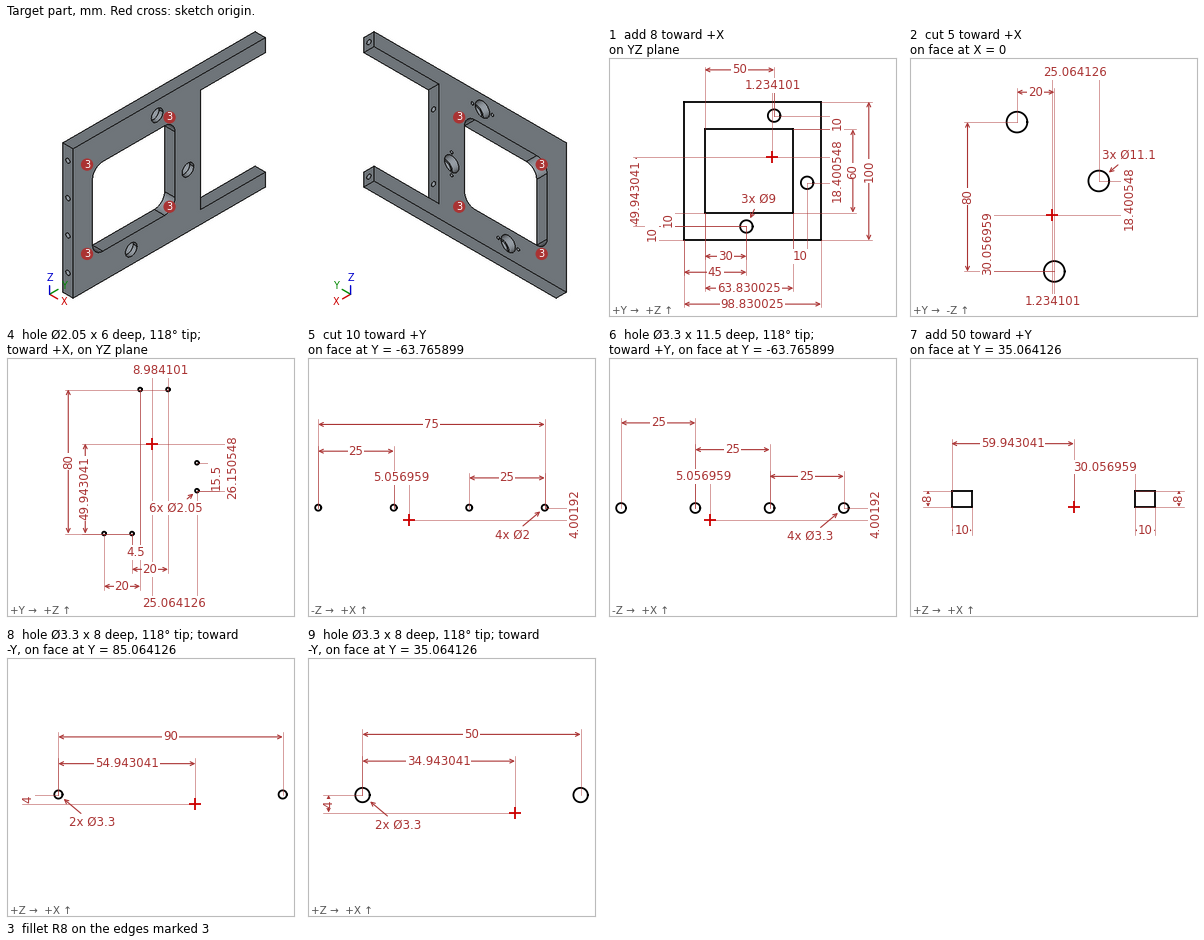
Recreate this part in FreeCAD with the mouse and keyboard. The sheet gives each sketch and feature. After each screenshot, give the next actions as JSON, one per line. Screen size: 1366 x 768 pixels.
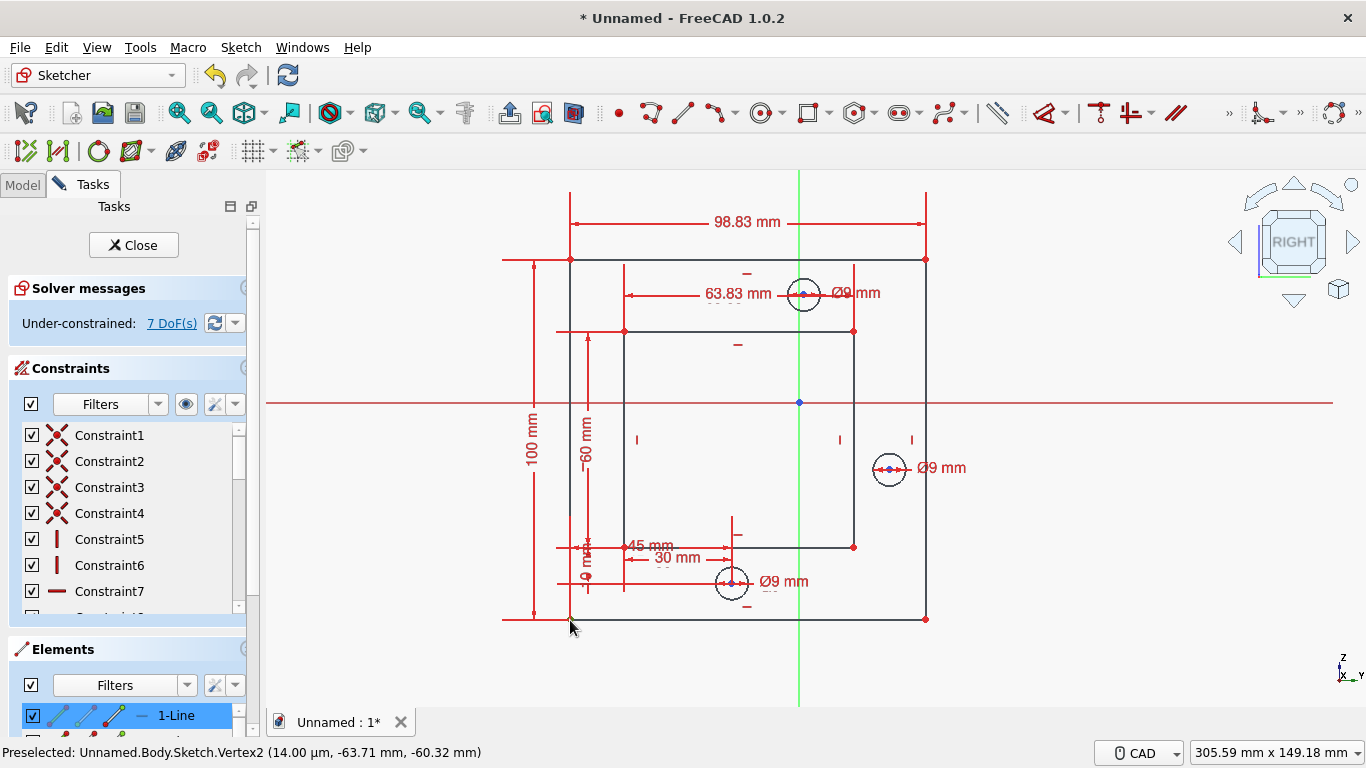
{"action": "left_click", "coordinate": [732, 584]}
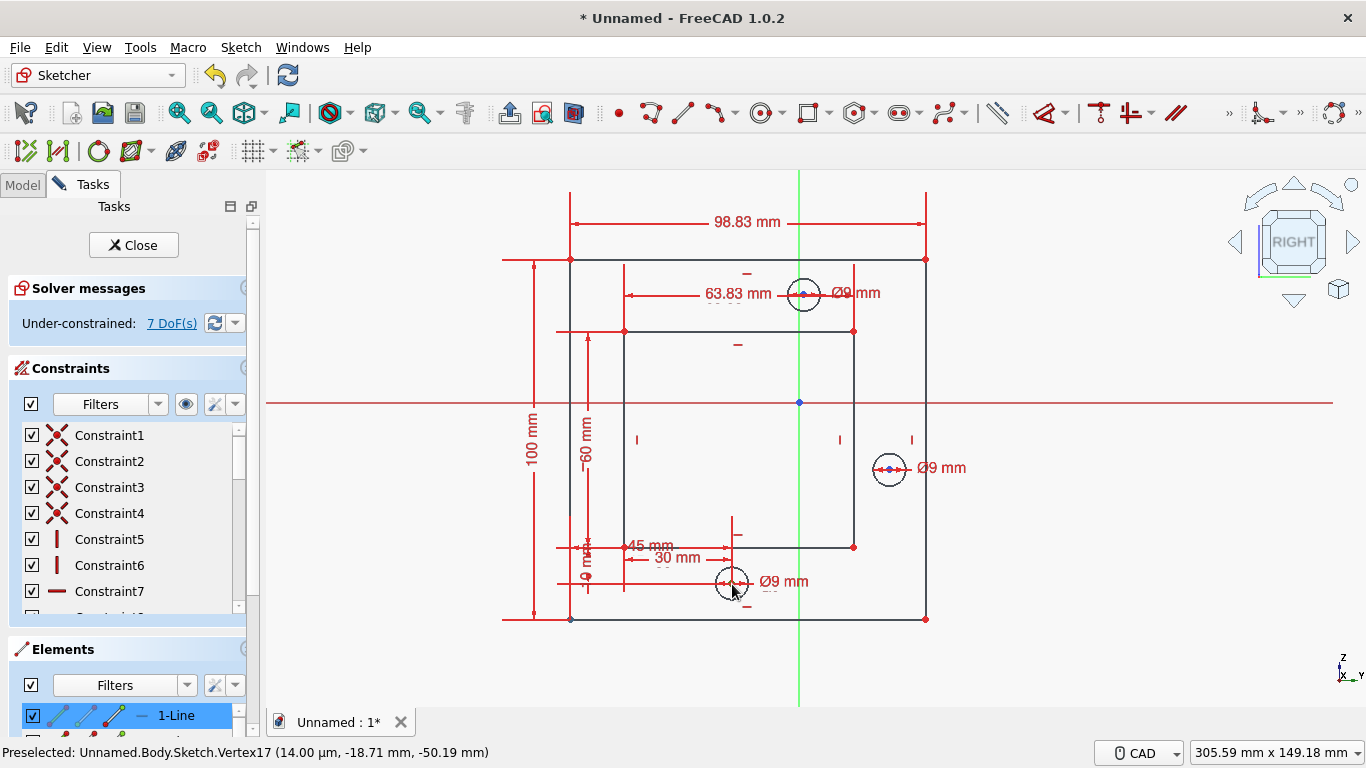
{"action": "key", "text": "i"}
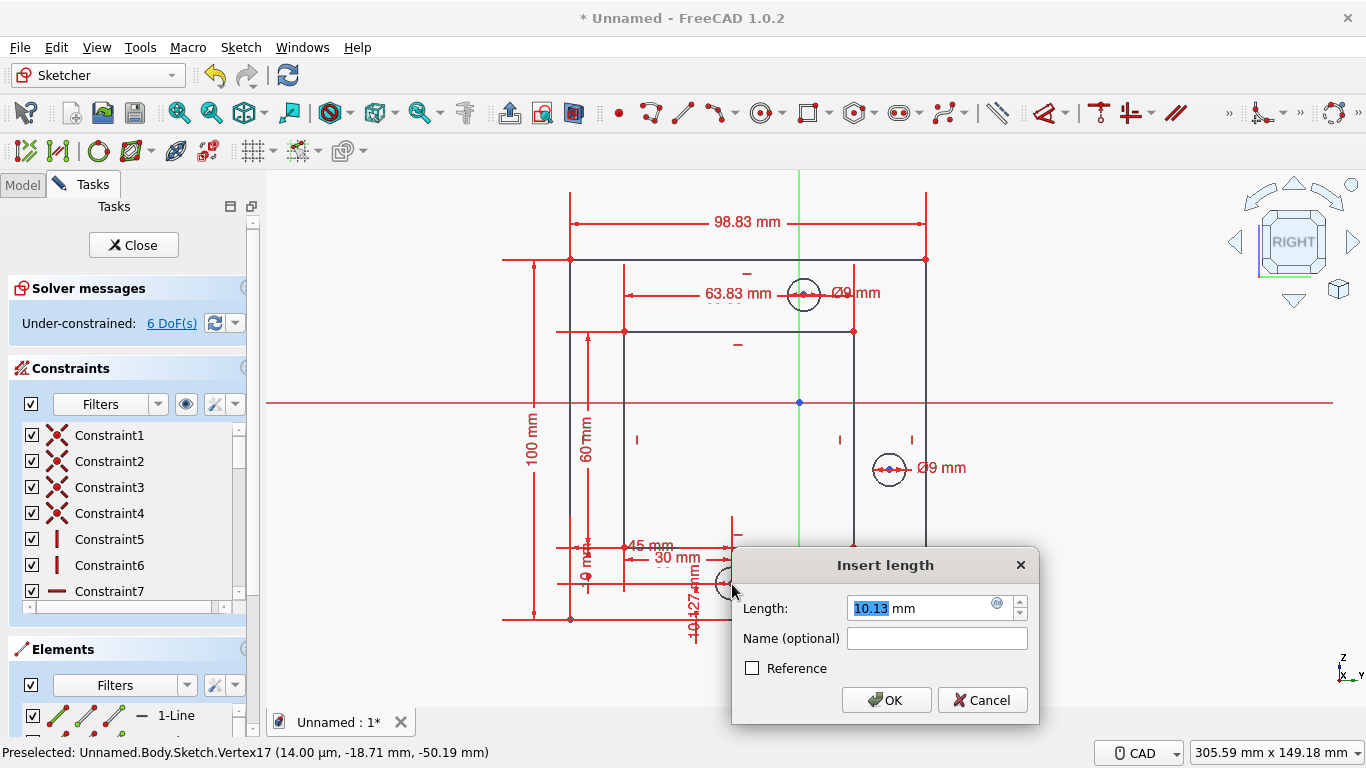
{"action": "type", "text": "10"}
{"action": "key", "text": "Return"}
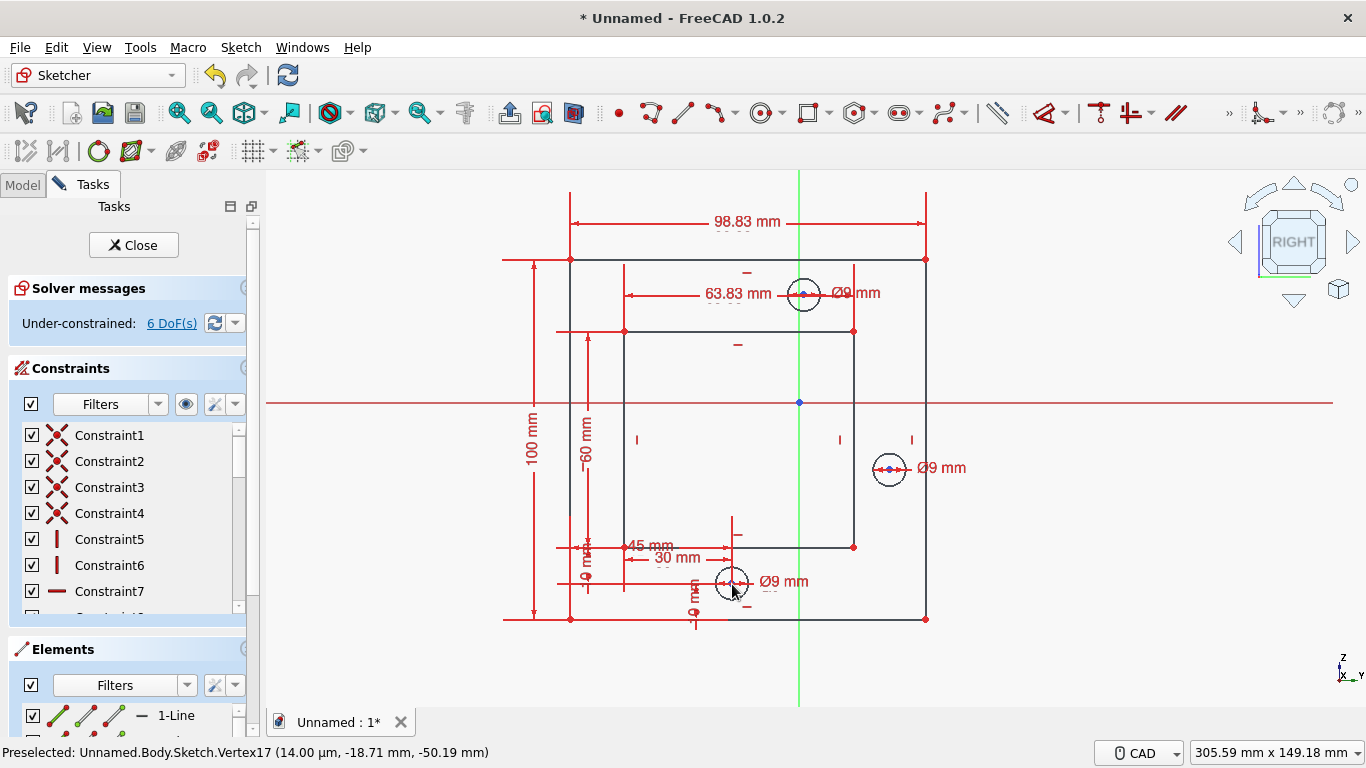
{"action": "left_click", "coordinate": [624, 332]}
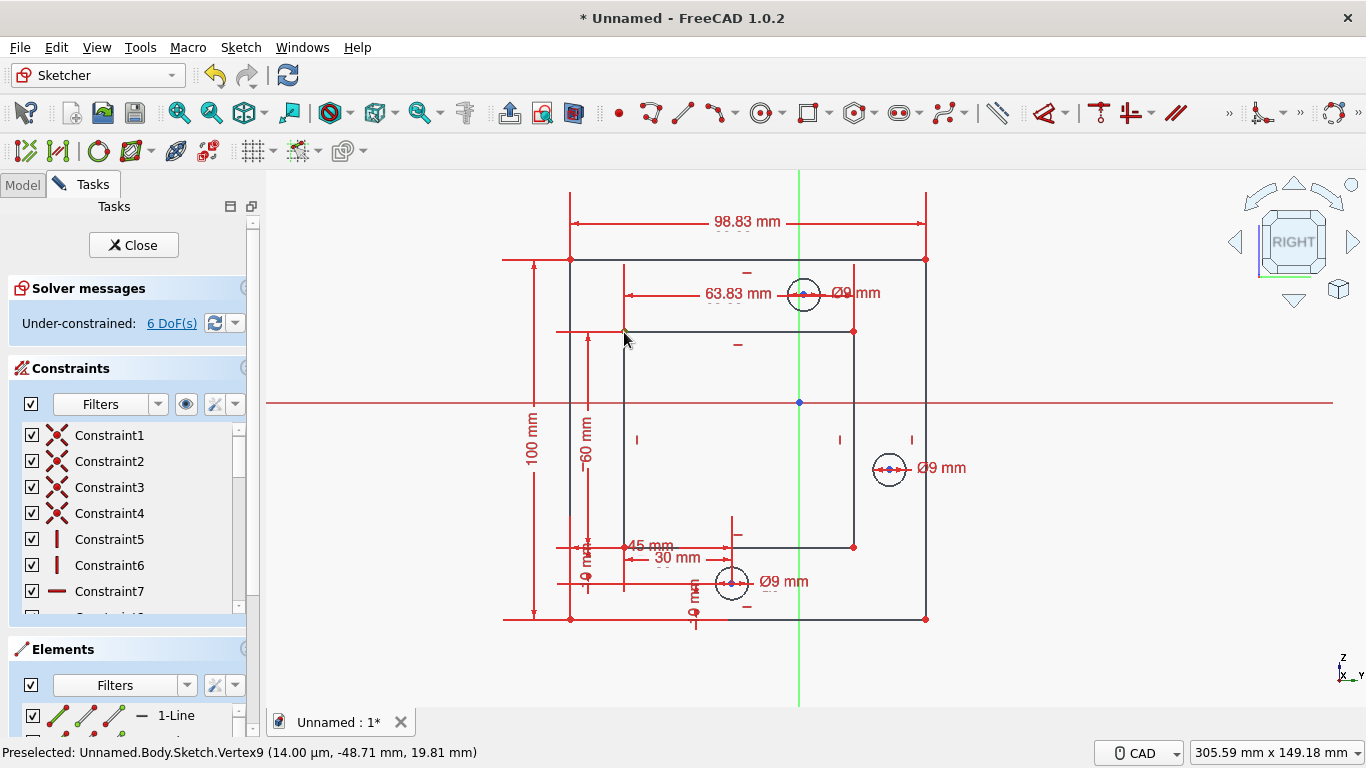
{"action": "left_click", "coordinate": [804, 295]}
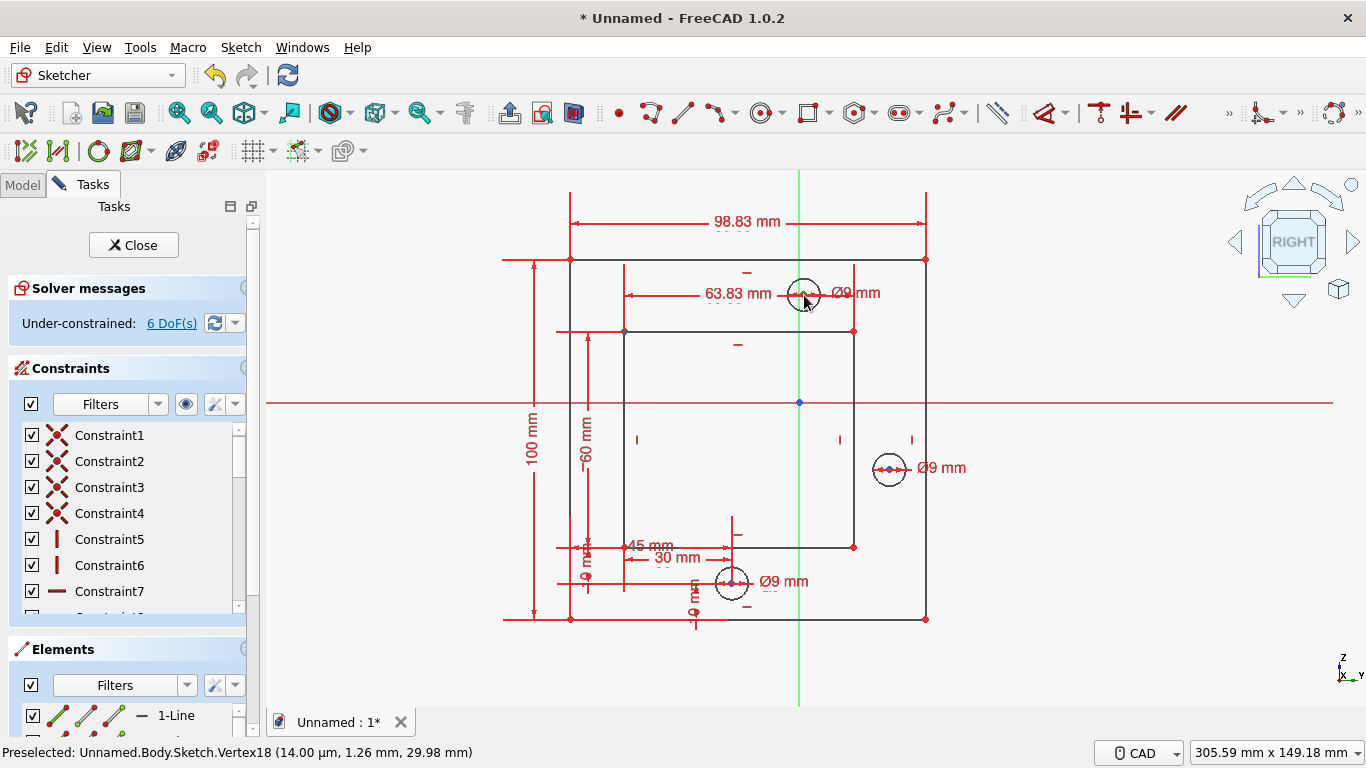
{"action": "left_click", "coordinate": [1068, 114]}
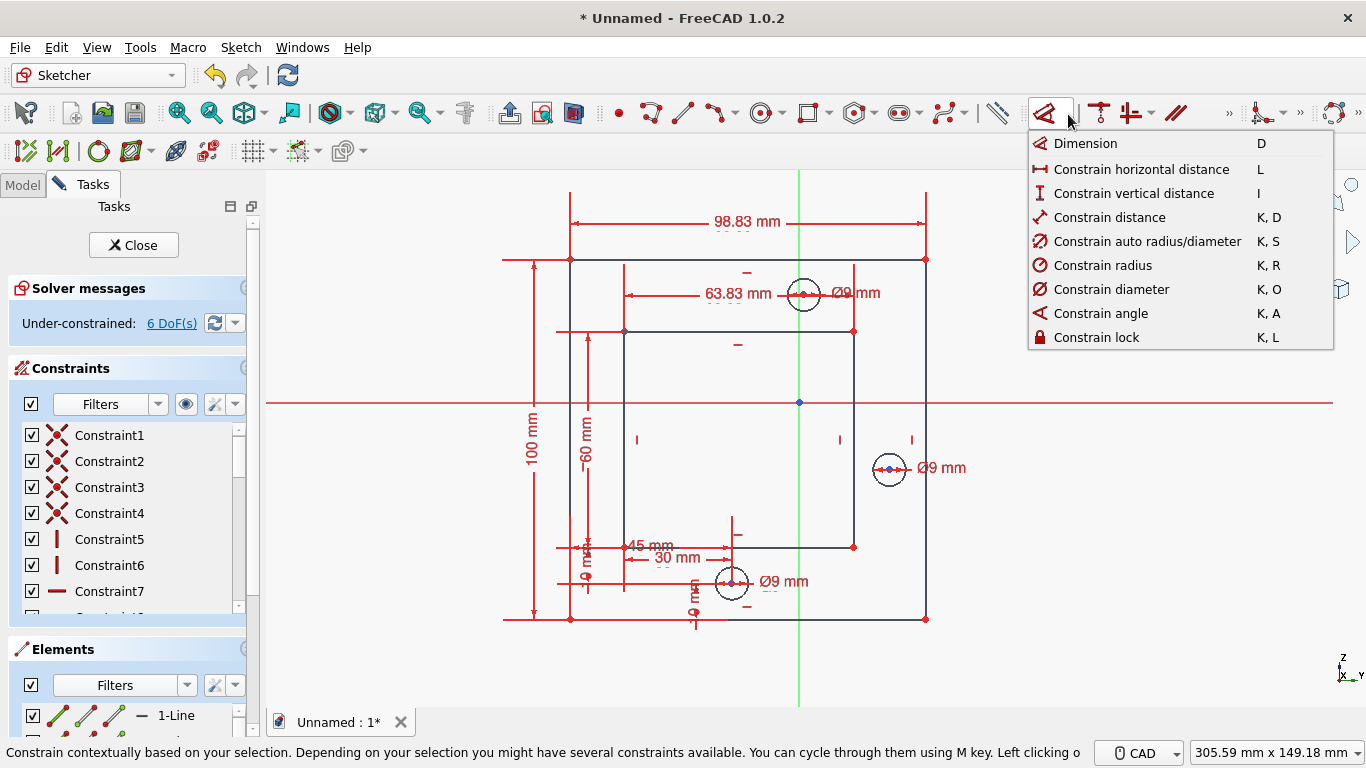
{"action": "left_click", "coordinate": [1181, 169]}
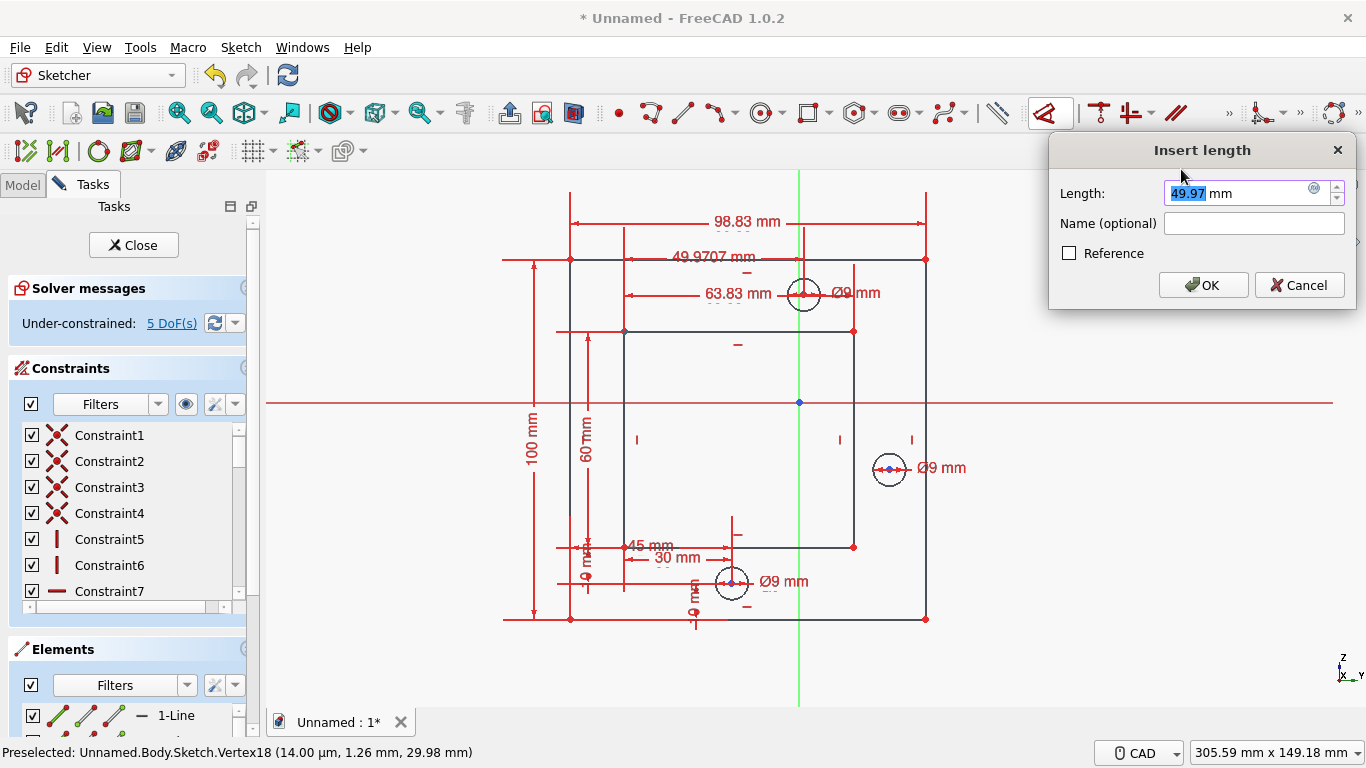
{"action": "type", "text": "50"}
{"action": "key", "text": "Return"}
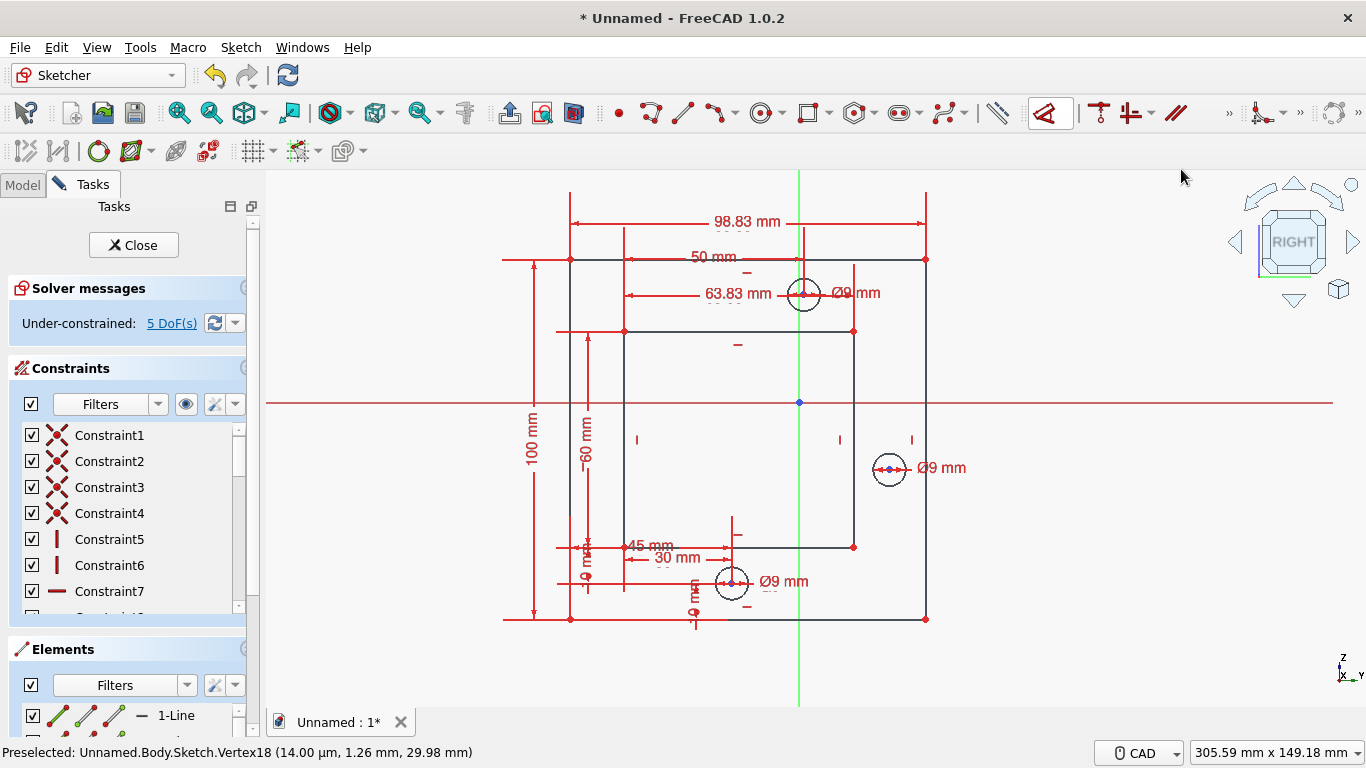
{"action": "left_click", "coordinate": [854, 332]}